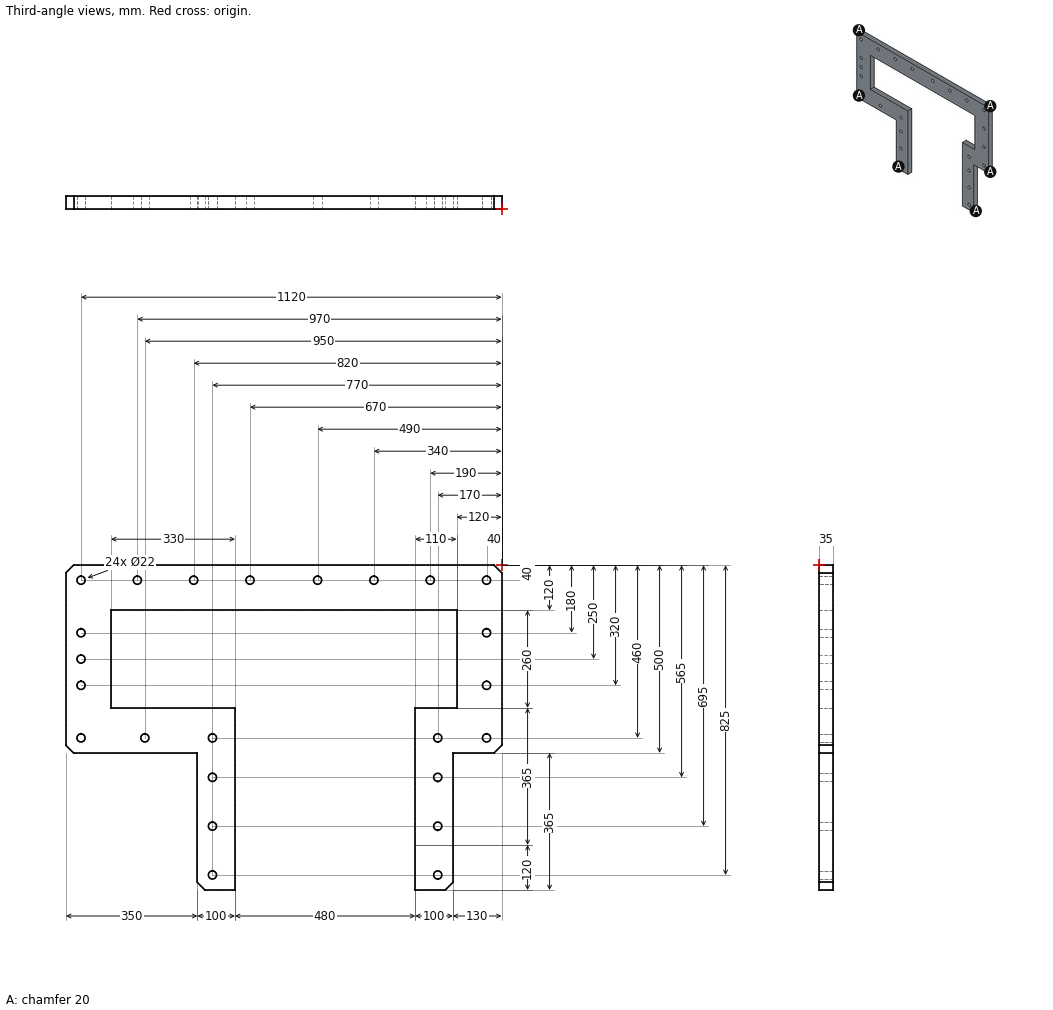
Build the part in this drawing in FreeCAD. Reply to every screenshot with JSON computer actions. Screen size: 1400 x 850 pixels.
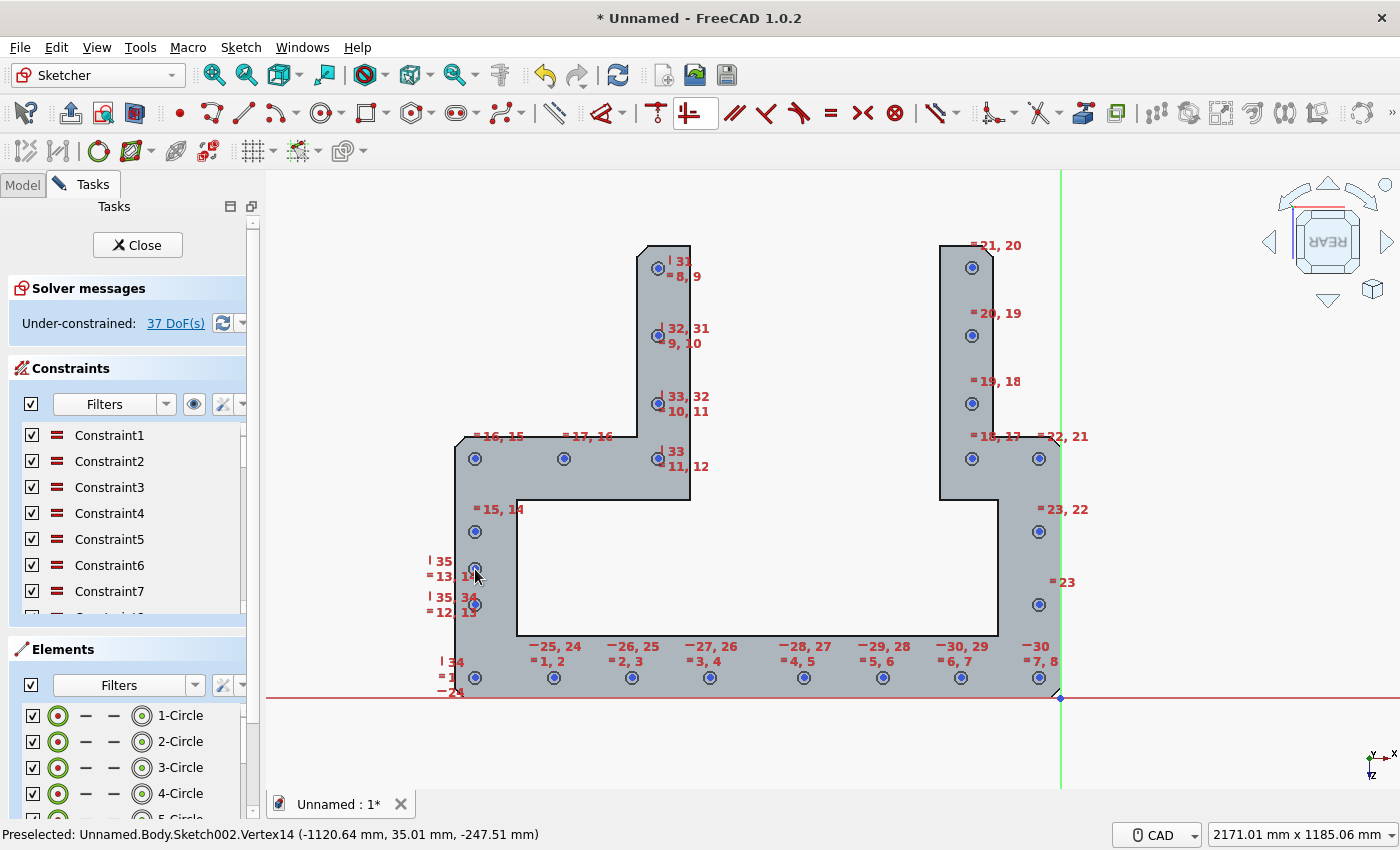
{"action": "left_click", "coordinate": [477, 571]}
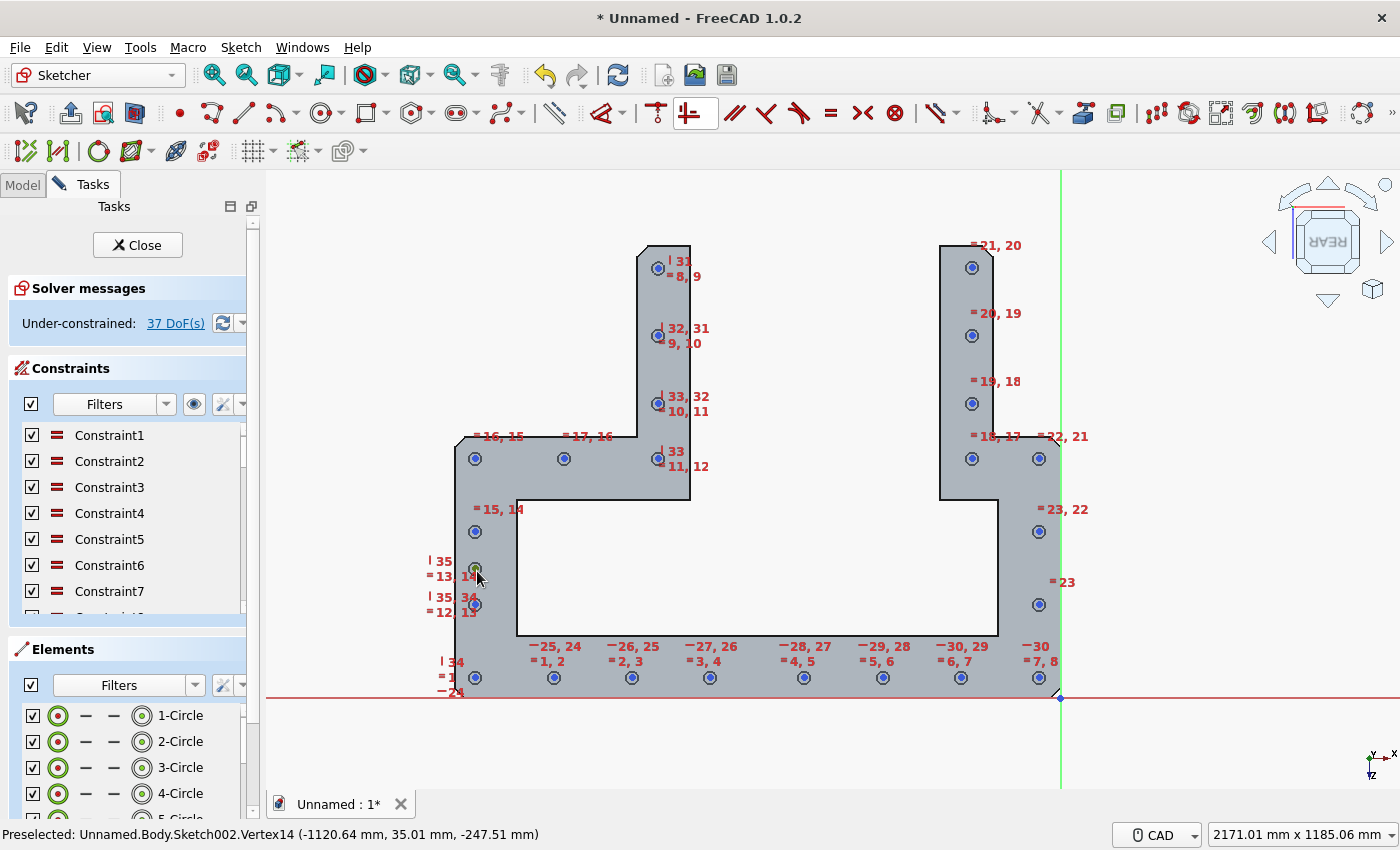
{"action": "left_click", "coordinate": [475, 532]}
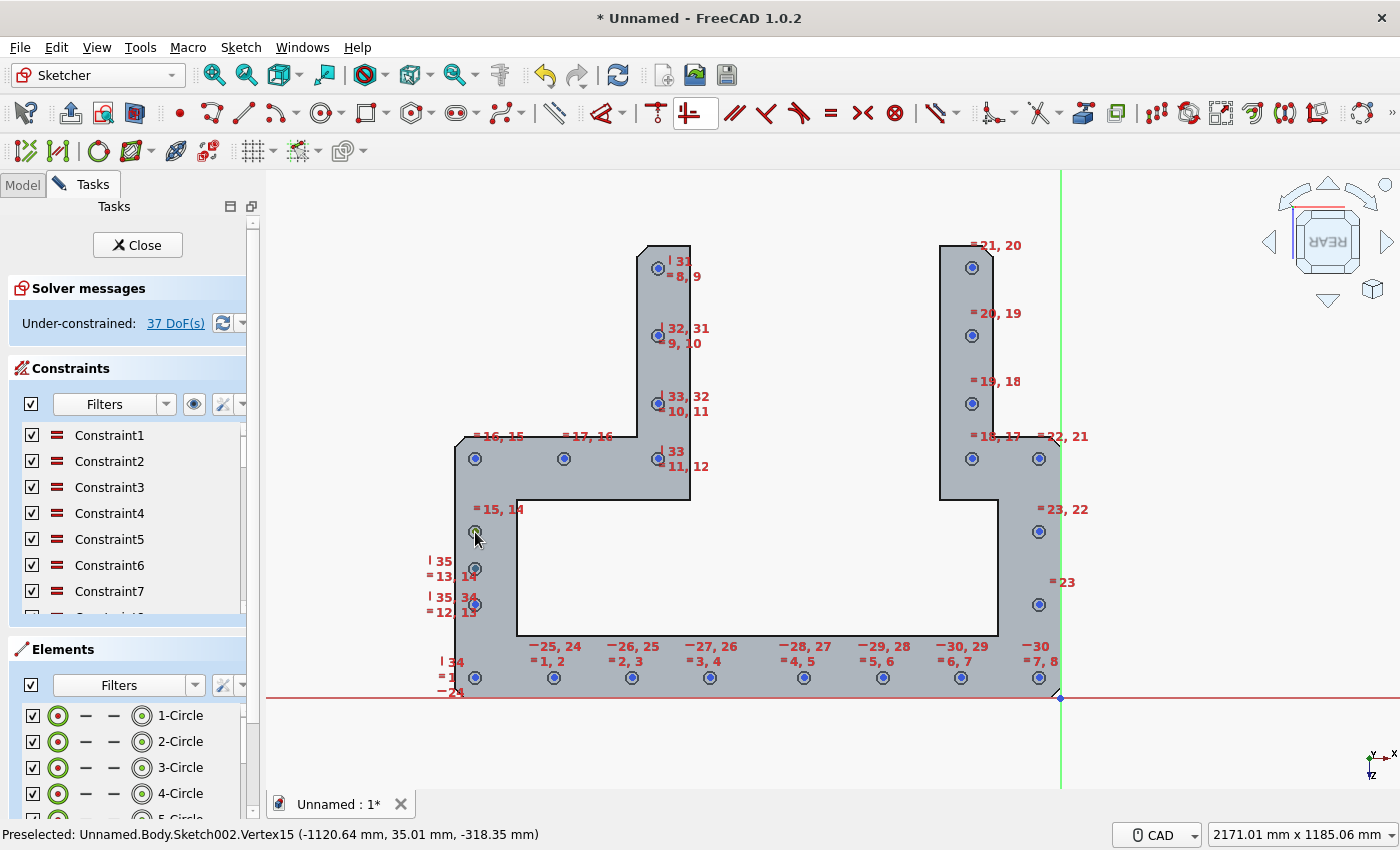
{"action": "key", "text": "v"}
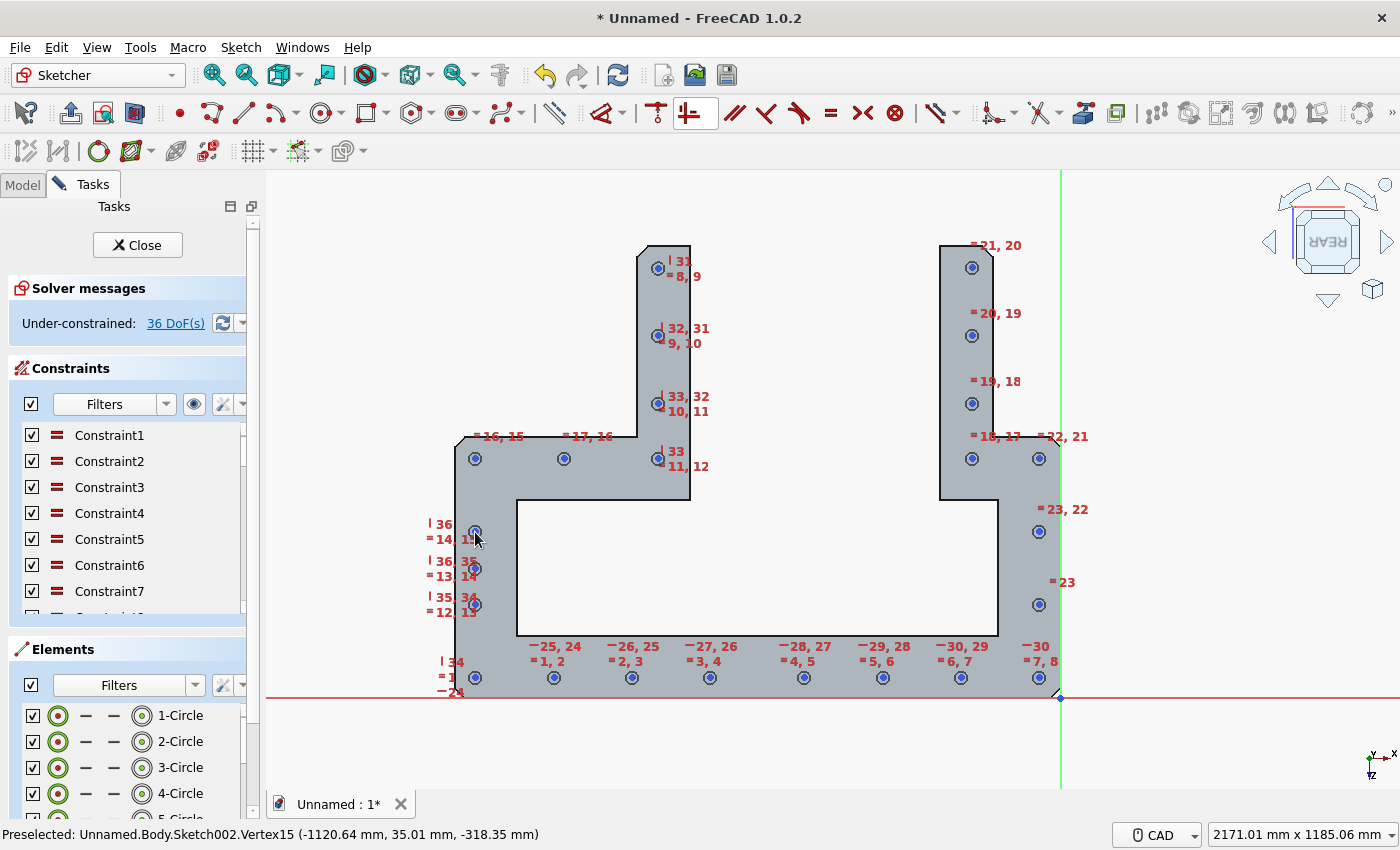
{"action": "left_click", "coordinate": [477, 534]}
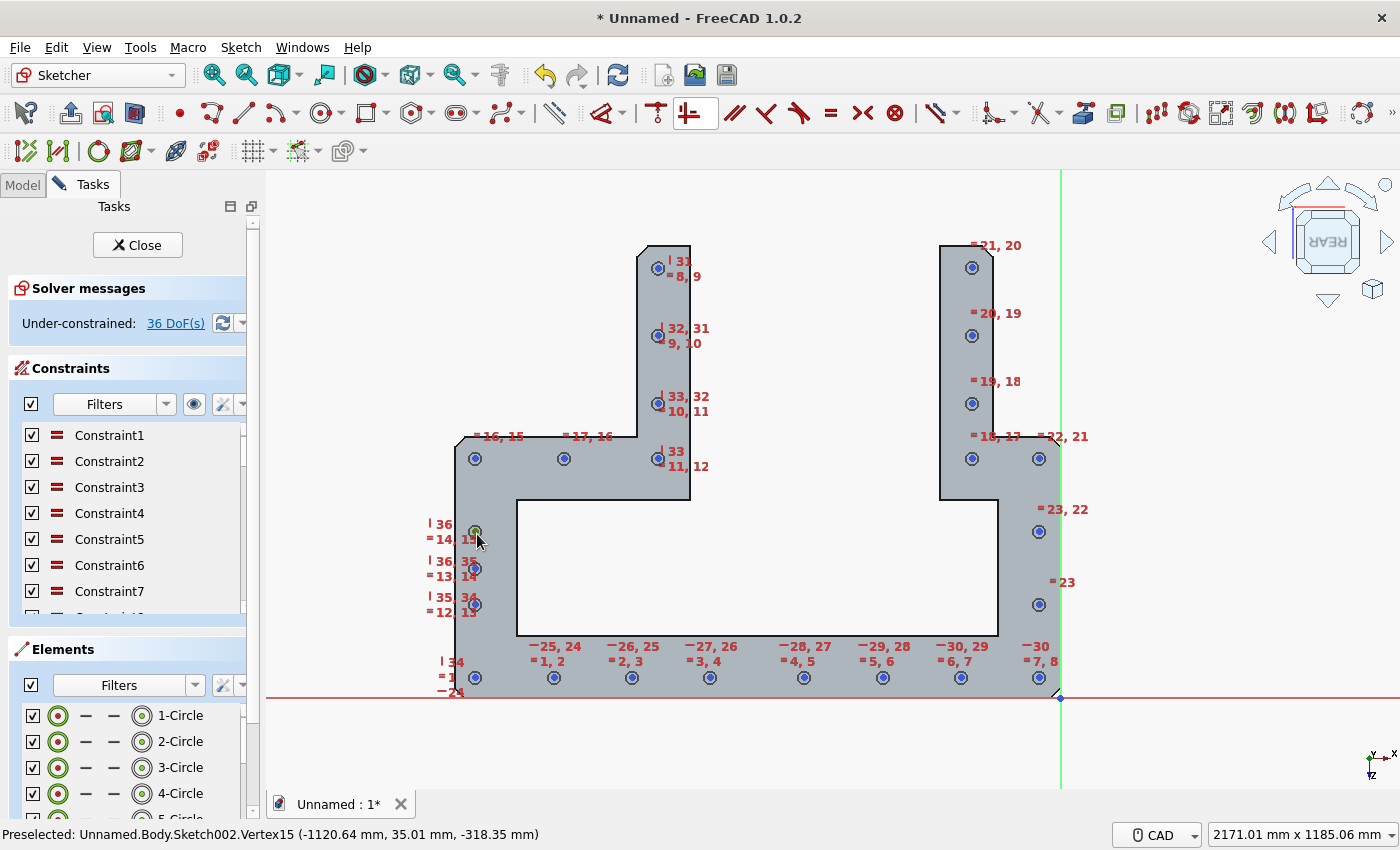
{"action": "left_click", "coordinate": [475, 459]}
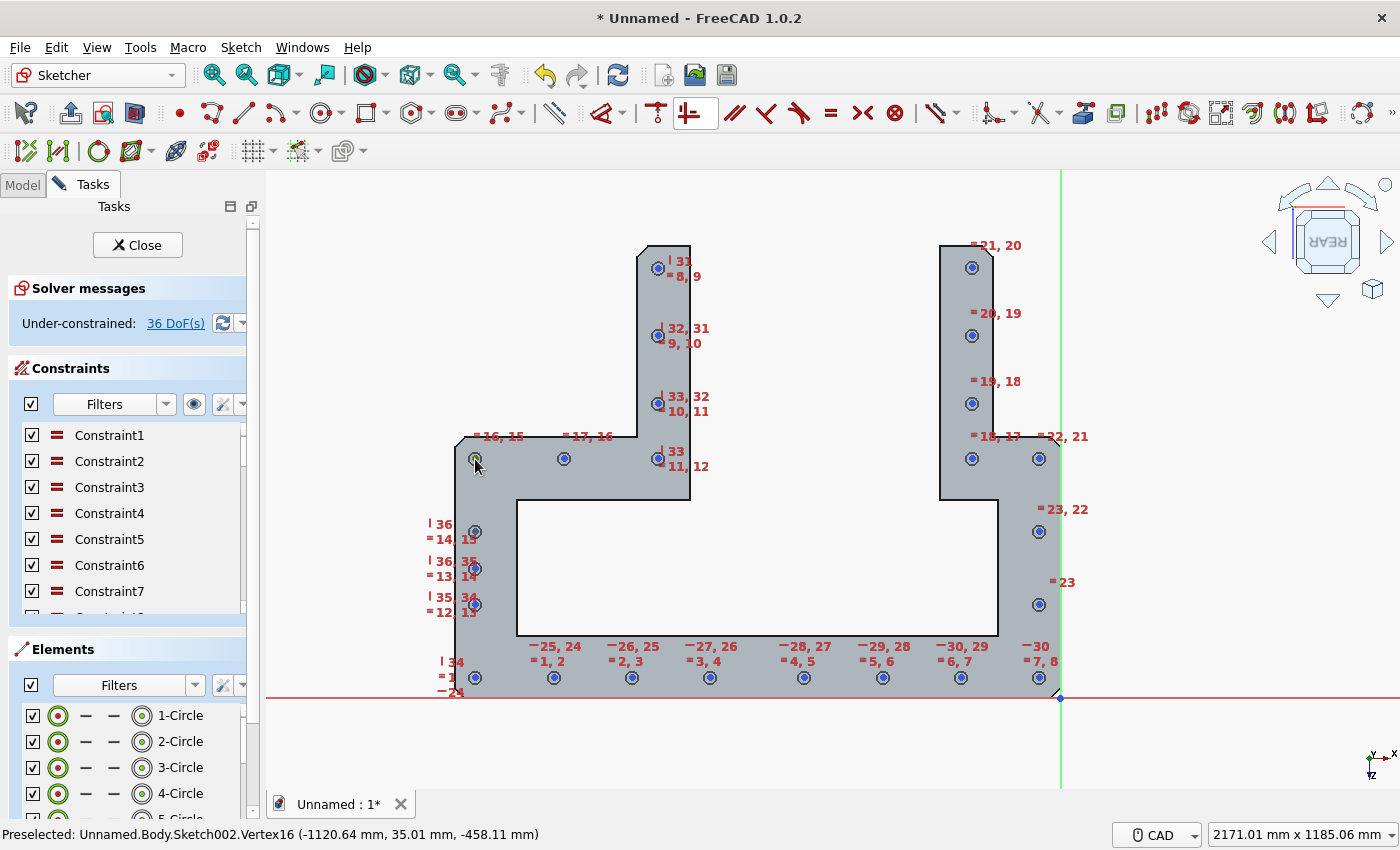
{"action": "key", "text": "v"}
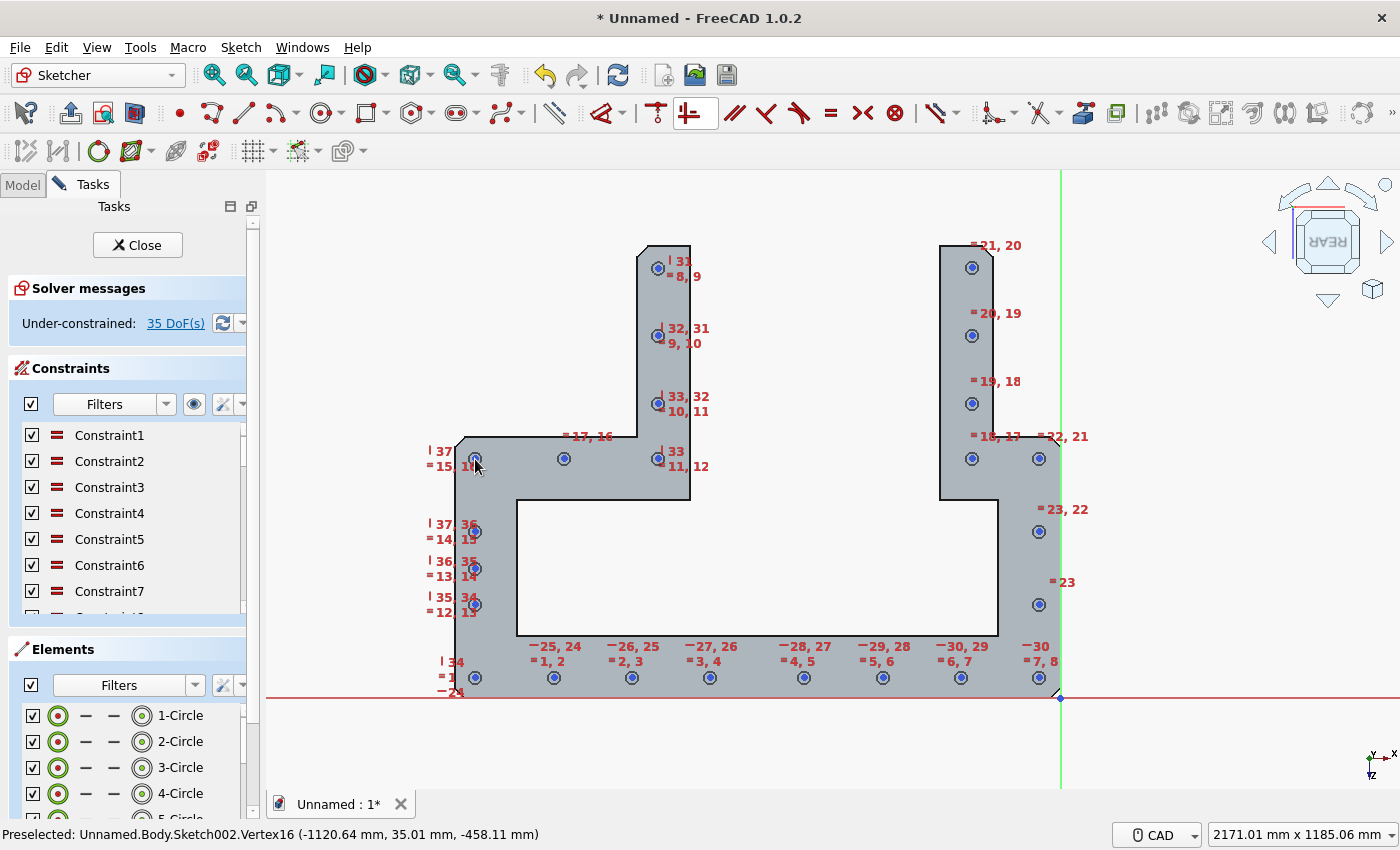
{"action": "left_click", "coordinate": [656, 461]}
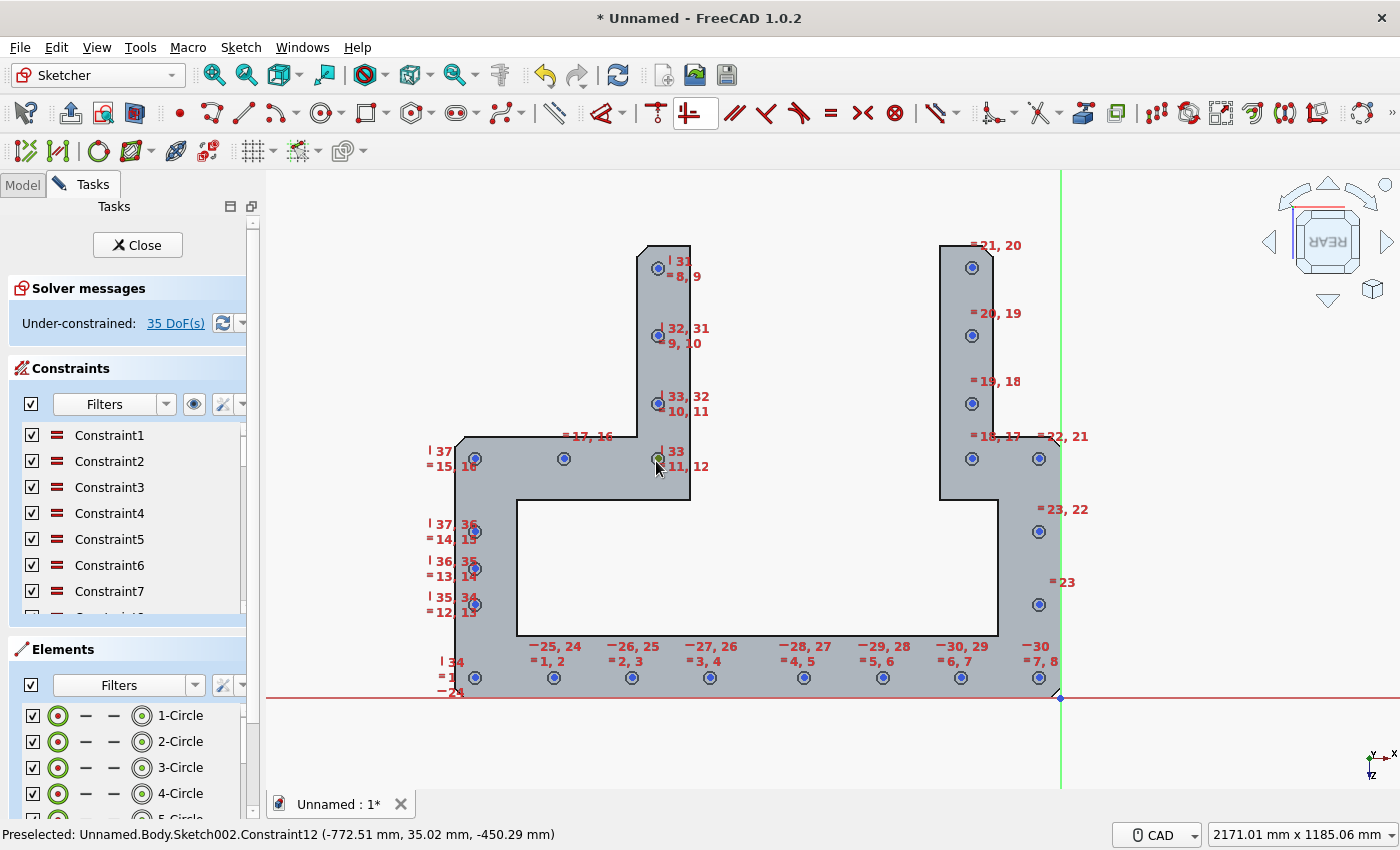
{"action": "left_click", "coordinate": [477, 461]}